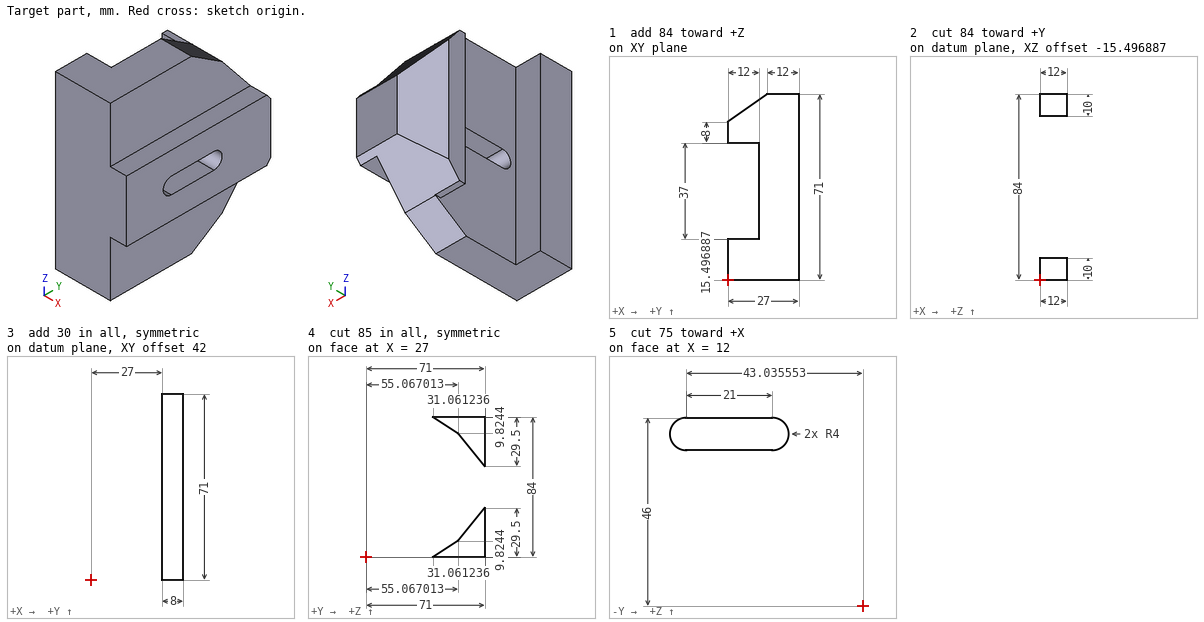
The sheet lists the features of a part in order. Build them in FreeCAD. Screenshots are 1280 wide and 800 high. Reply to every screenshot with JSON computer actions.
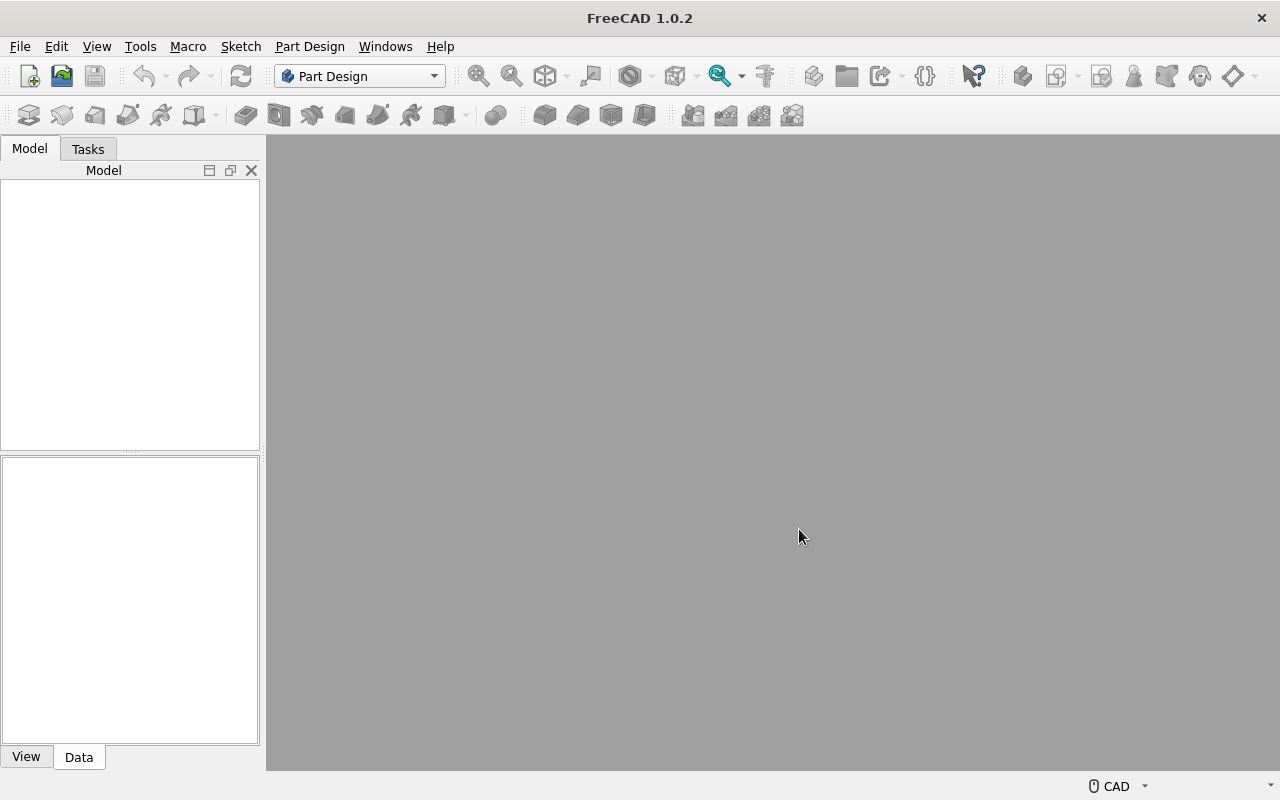
{"action": "left_click", "coordinate": [29, 76]}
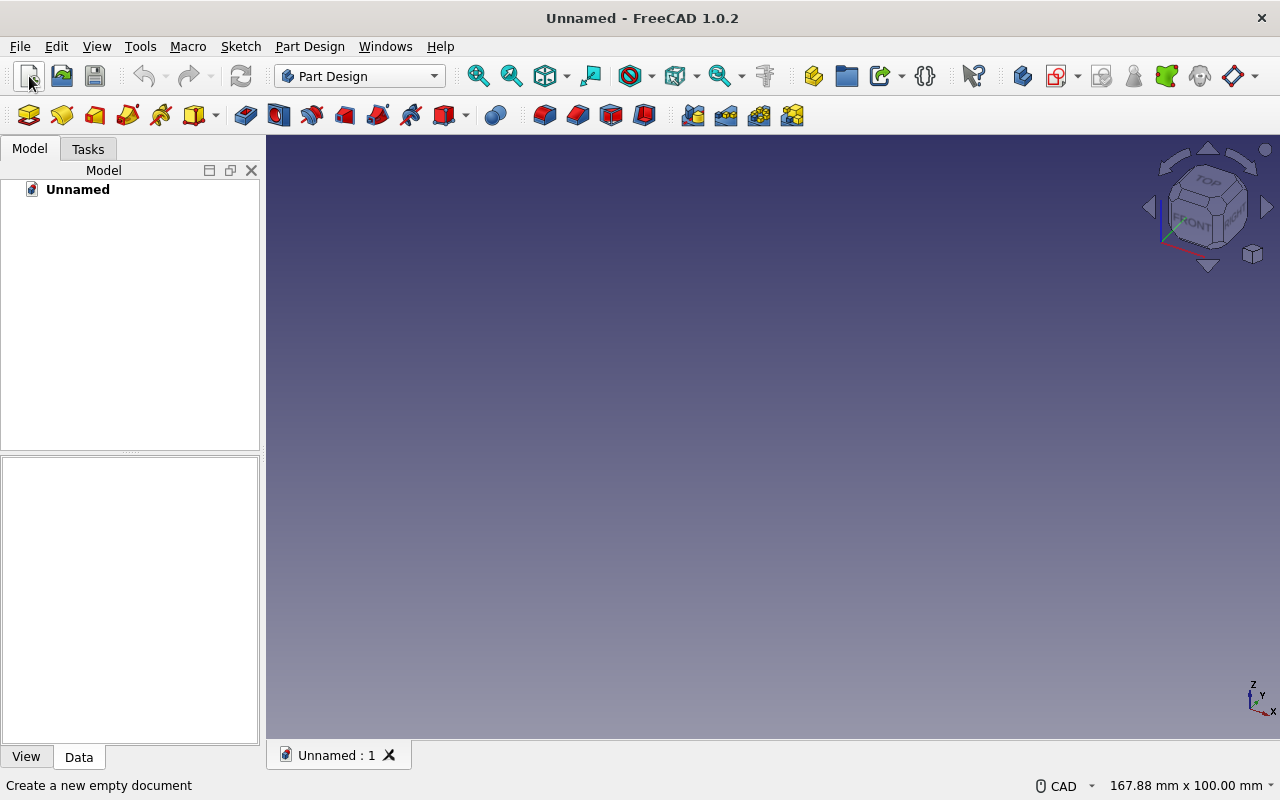
{"action": "left_click", "coordinate": [1056, 76]}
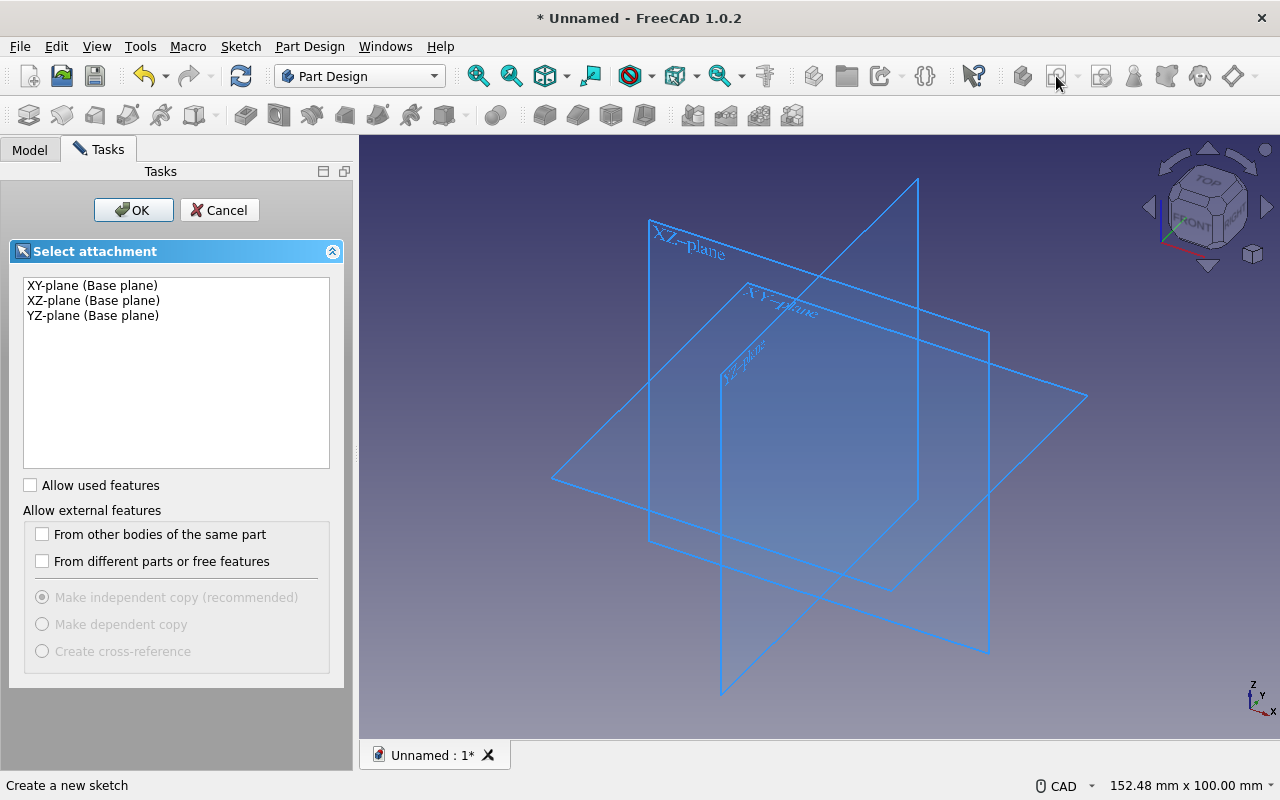
{"action": "left_click", "coordinate": [84, 286]}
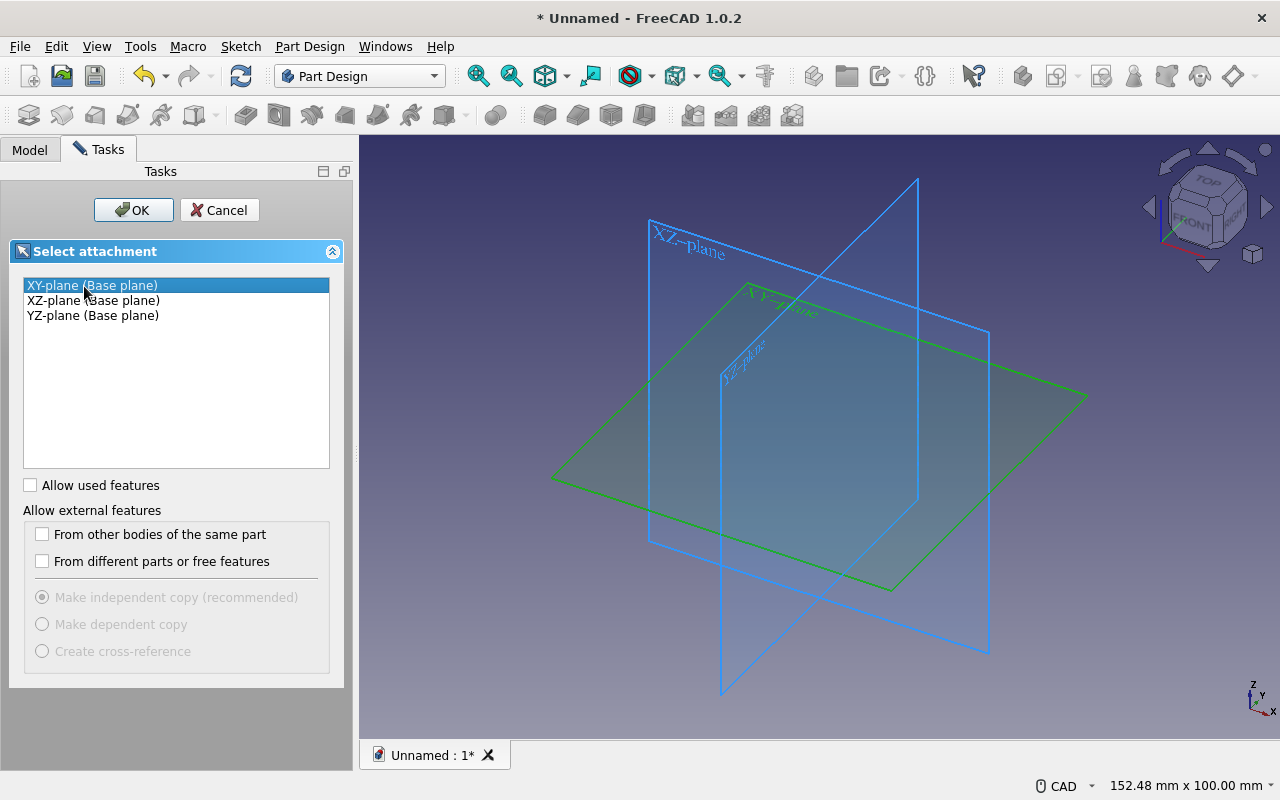
{"action": "left_click", "coordinate": [134, 210]}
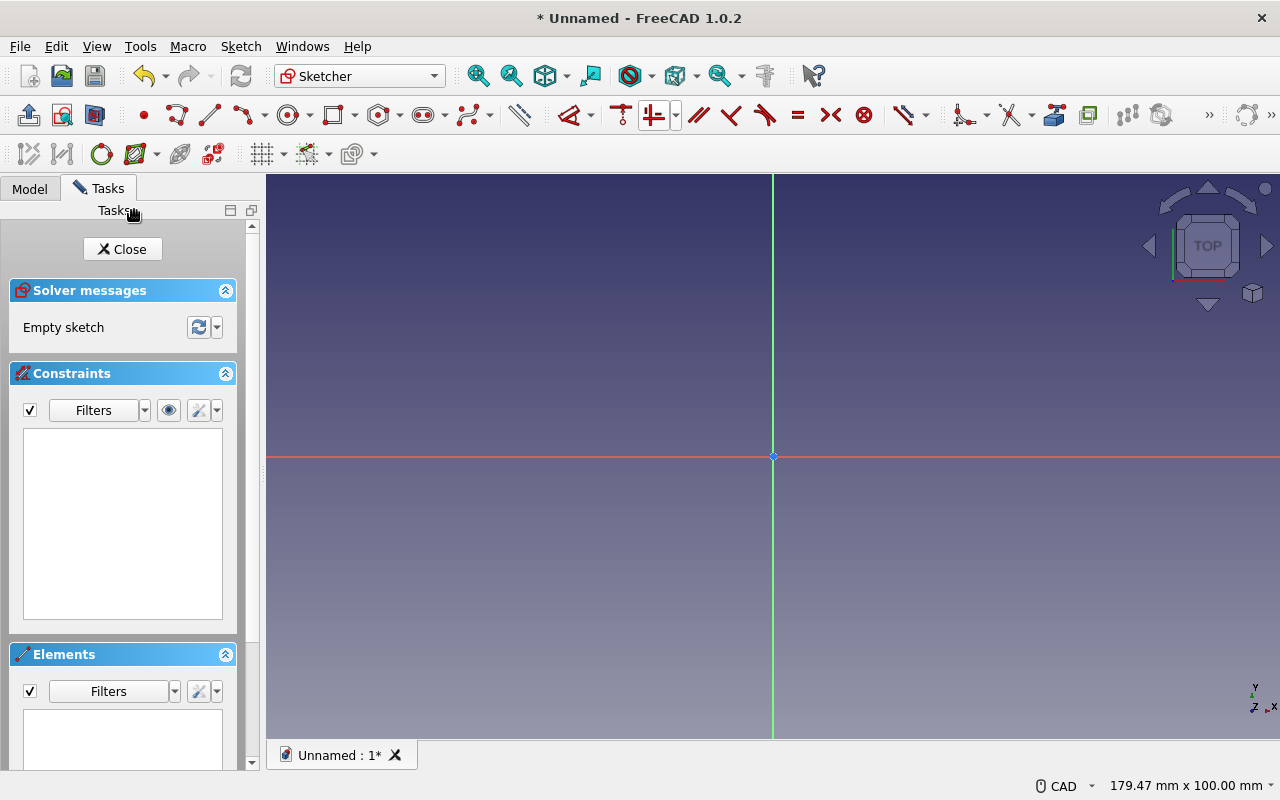
{"action": "scroll", "coordinate": [410, 711], "scroll_direction": "down", "scroll_amount": 2}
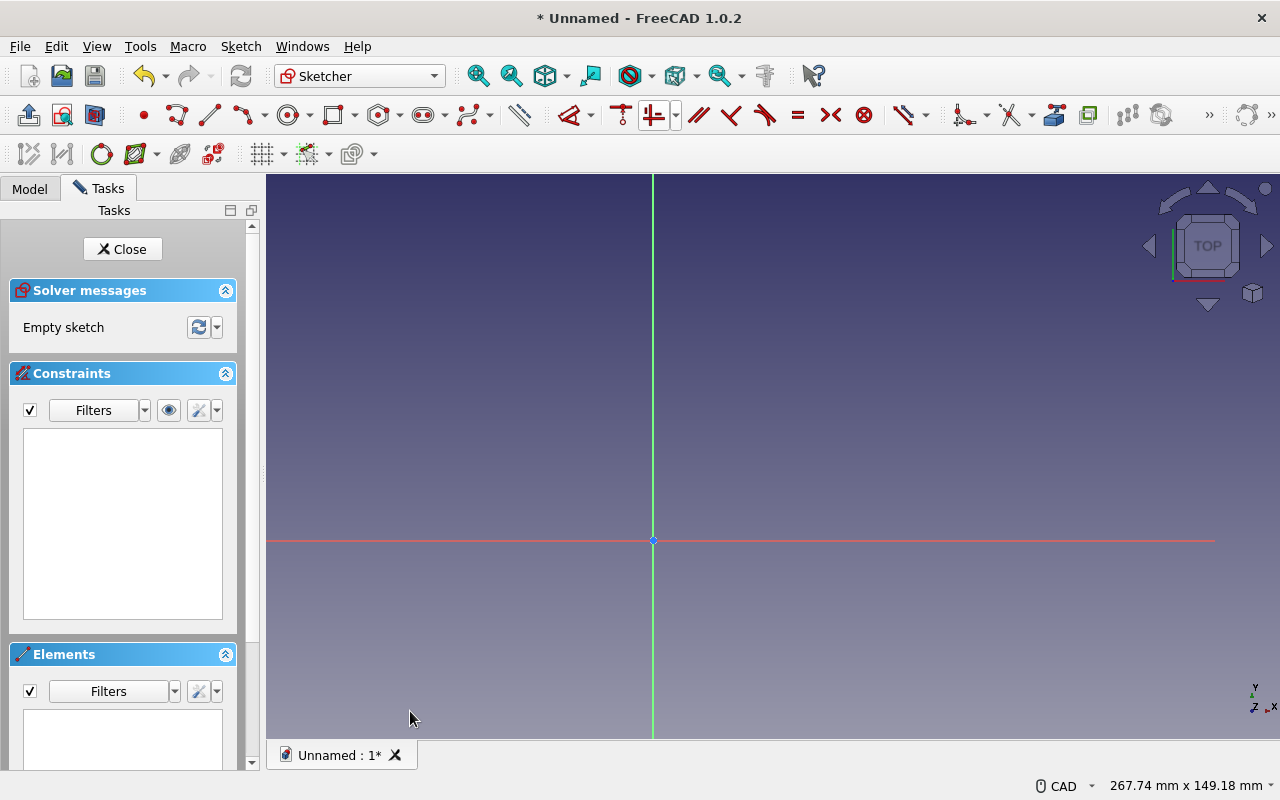
{"action": "left_click", "coordinate": [177, 116]}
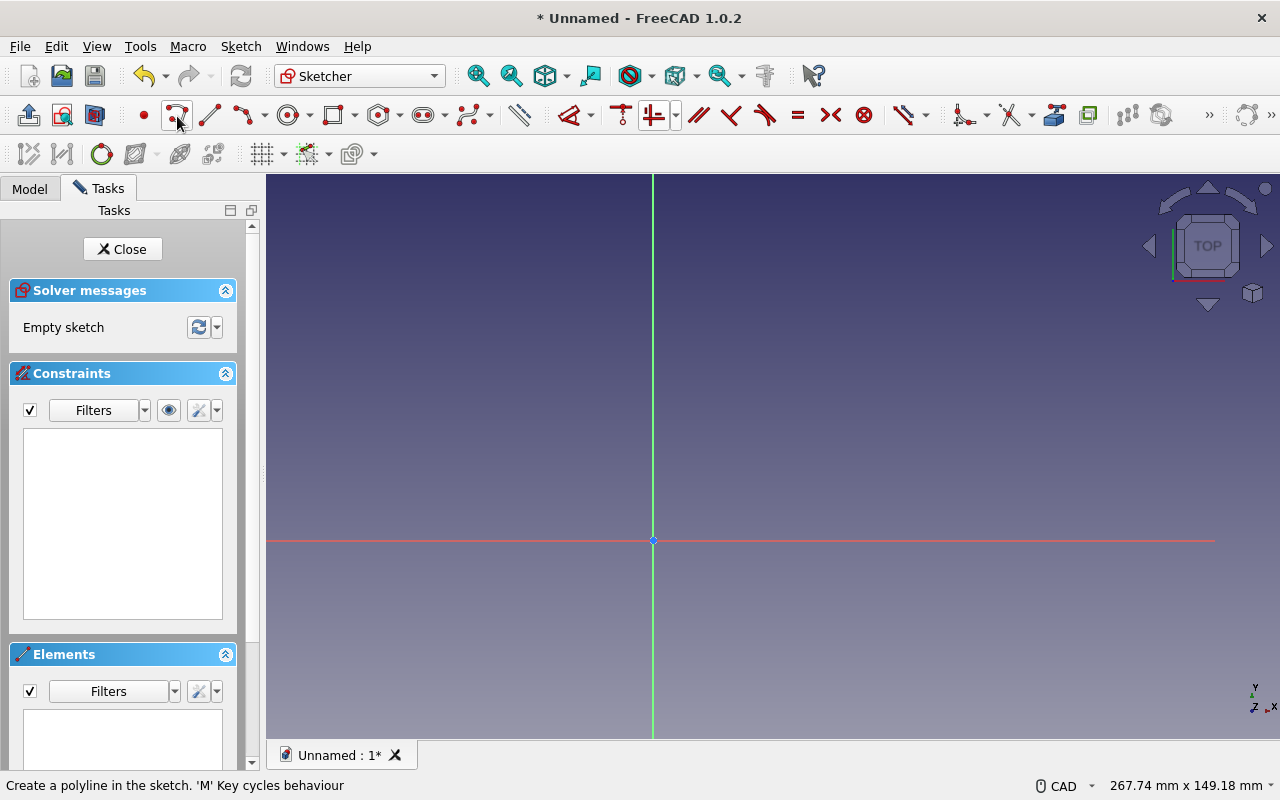
{"action": "left_click", "coordinate": [653, 541]}
{"action": "left_click", "coordinate": [756, 532]}
{"action": "left_click", "coordinate": [756, 272]}
{"action": "left_click", "coordinate": [710, 272]}
{"action": "left_click", "coordinate": [653, 312]}
{"action": "left_click", "coordinate": [662, 342]}
{"action": "left_click", "coordinate": [699, 342]}
{"action": "left_click", "coordinate": [699, 482]}
{"action": "left_click", "coordinate": [662, 482]}
{"action": "left_click", "coordinate": [653, 541]}
{"action": "key", "text": "Escape"}
{"action": "key", "text": "Escape"}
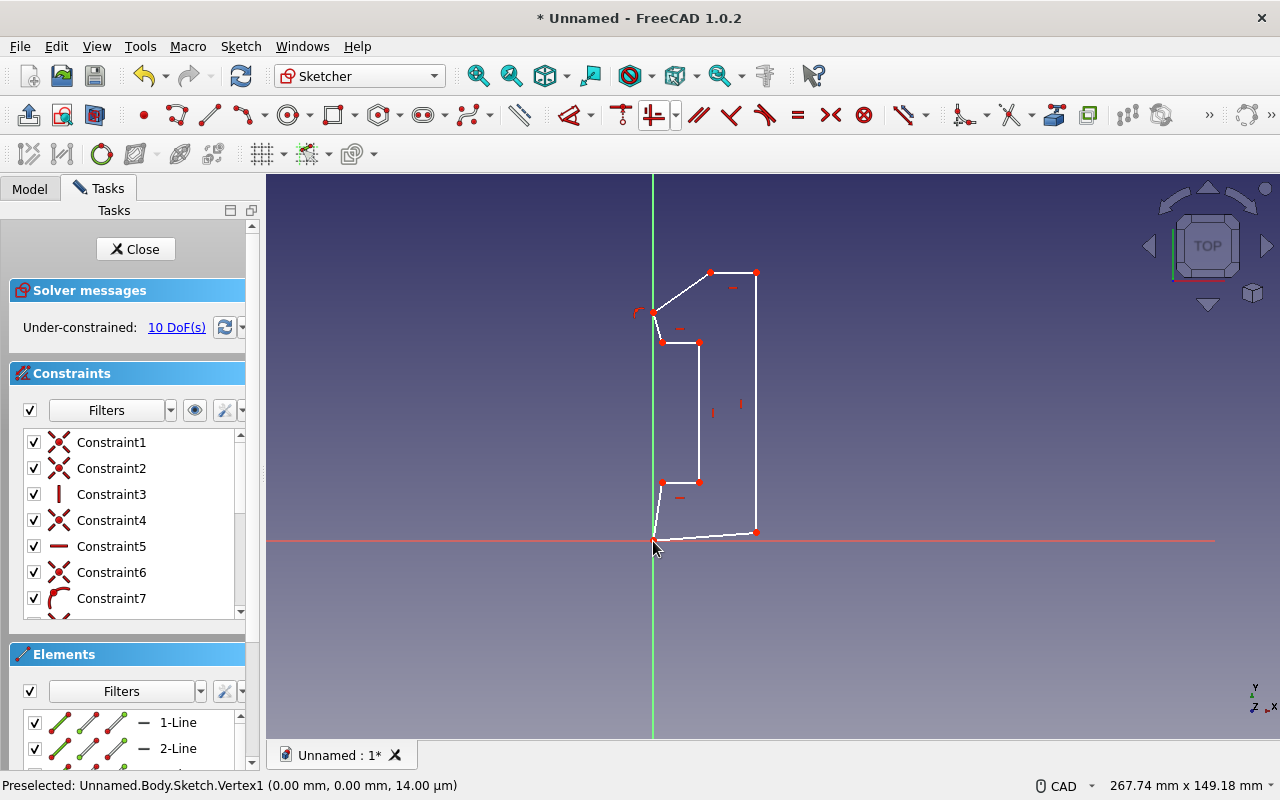
{"action": "left_click", "coordinate": [684, 538]}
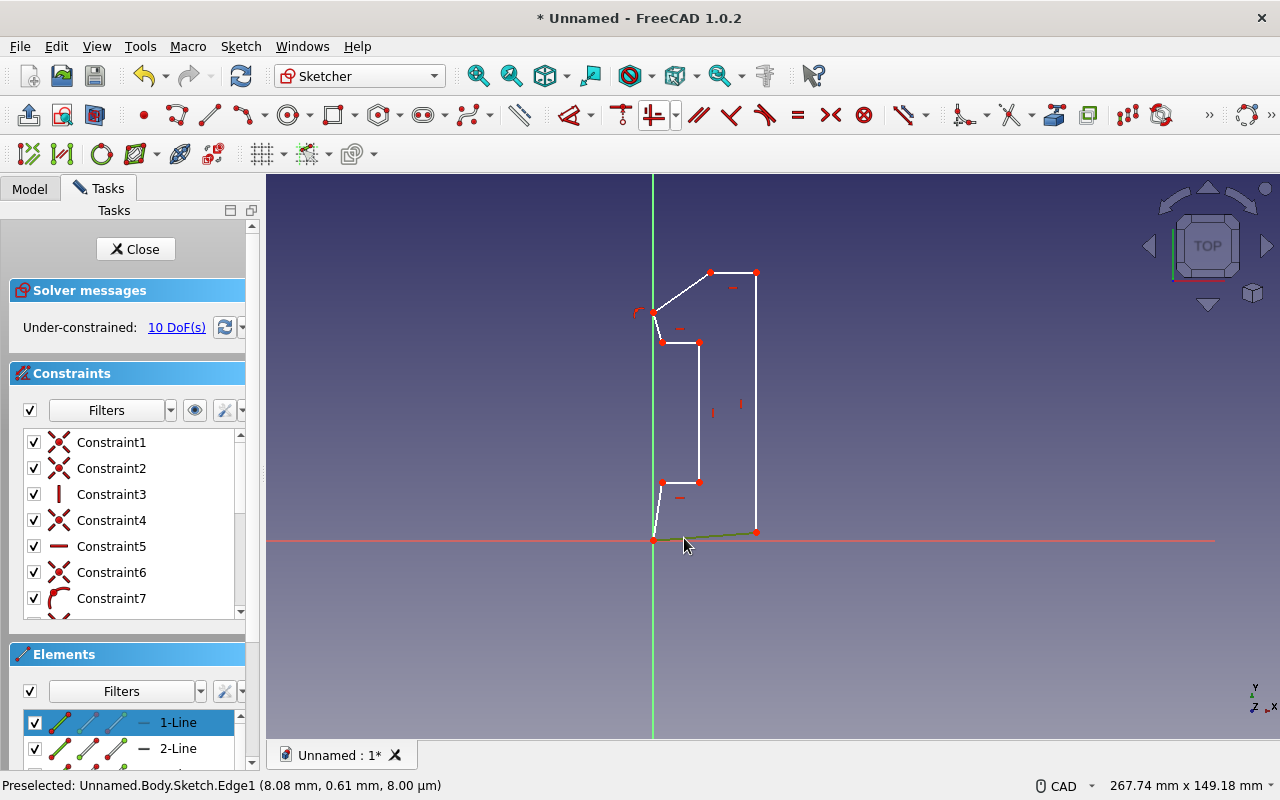
{"action": "key", "text": "h"}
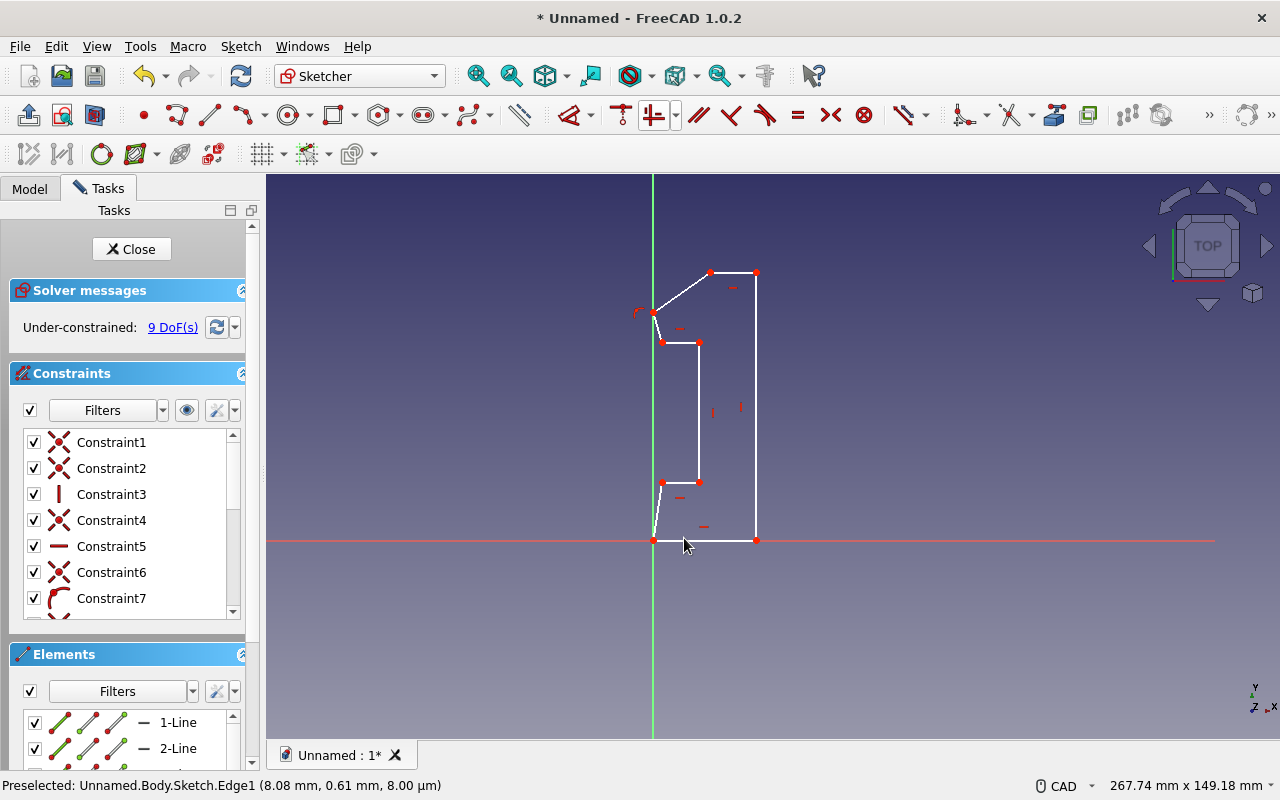
{"action": "scroll", "coordinate": [656, 322], "scroll_direction": "up", "scroll_amount": 2}